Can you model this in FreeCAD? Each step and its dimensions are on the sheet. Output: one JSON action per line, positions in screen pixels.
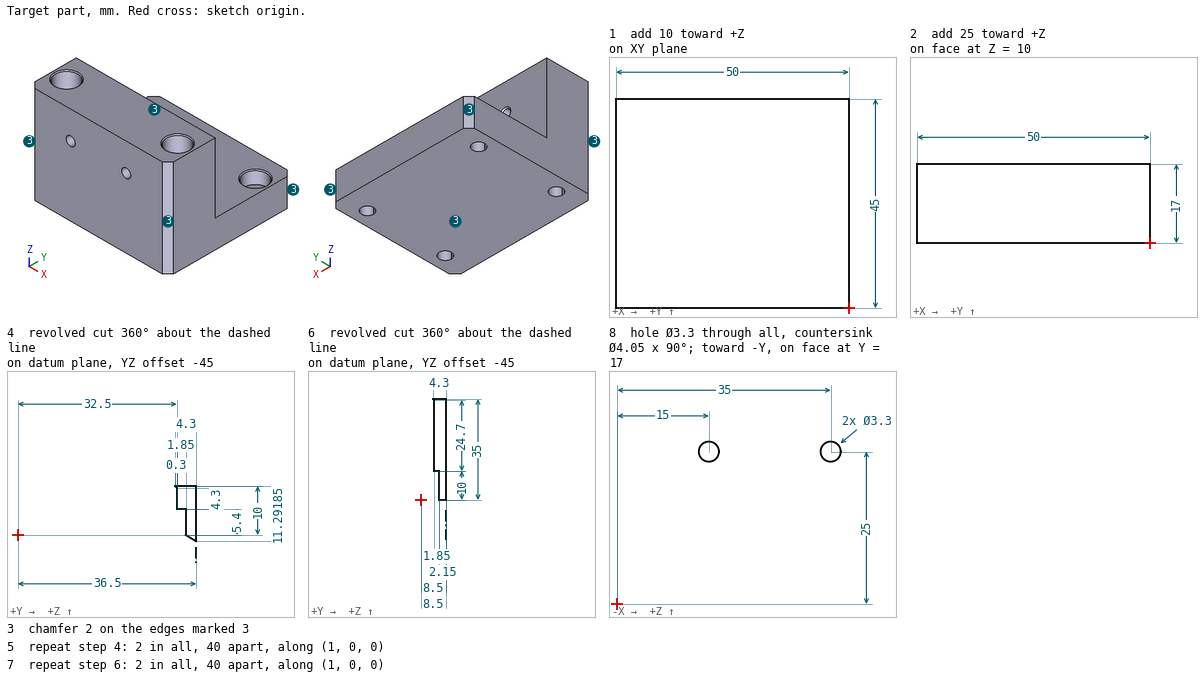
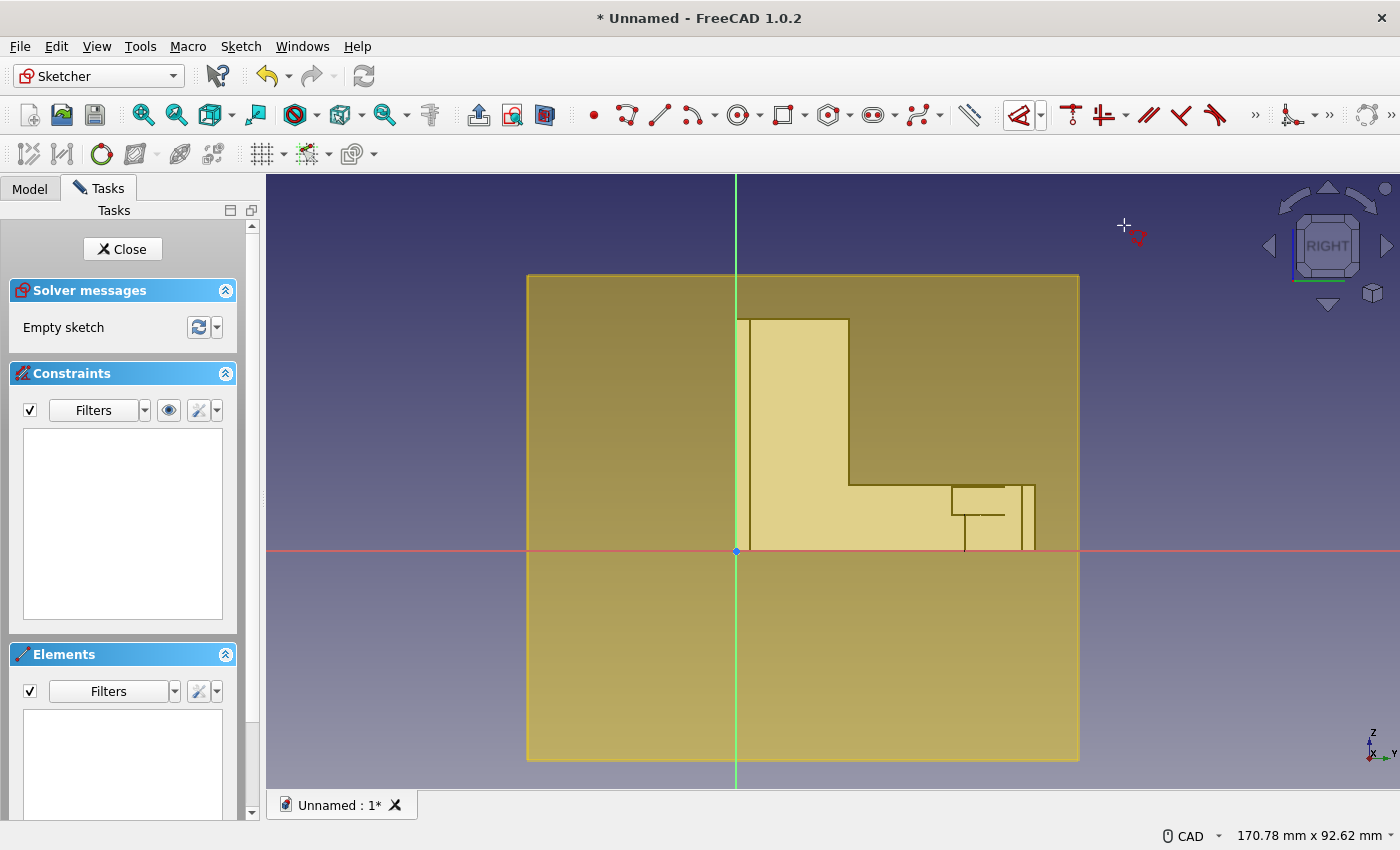
{"action": "left_click", "coordinate": [779, 551]}
{"action": "left_click", "coordinate": [793, 542]}
{"action": "left_click", "coordinate": [793, 319]}
{"action": "left_click", "coordinate": [764, 319]}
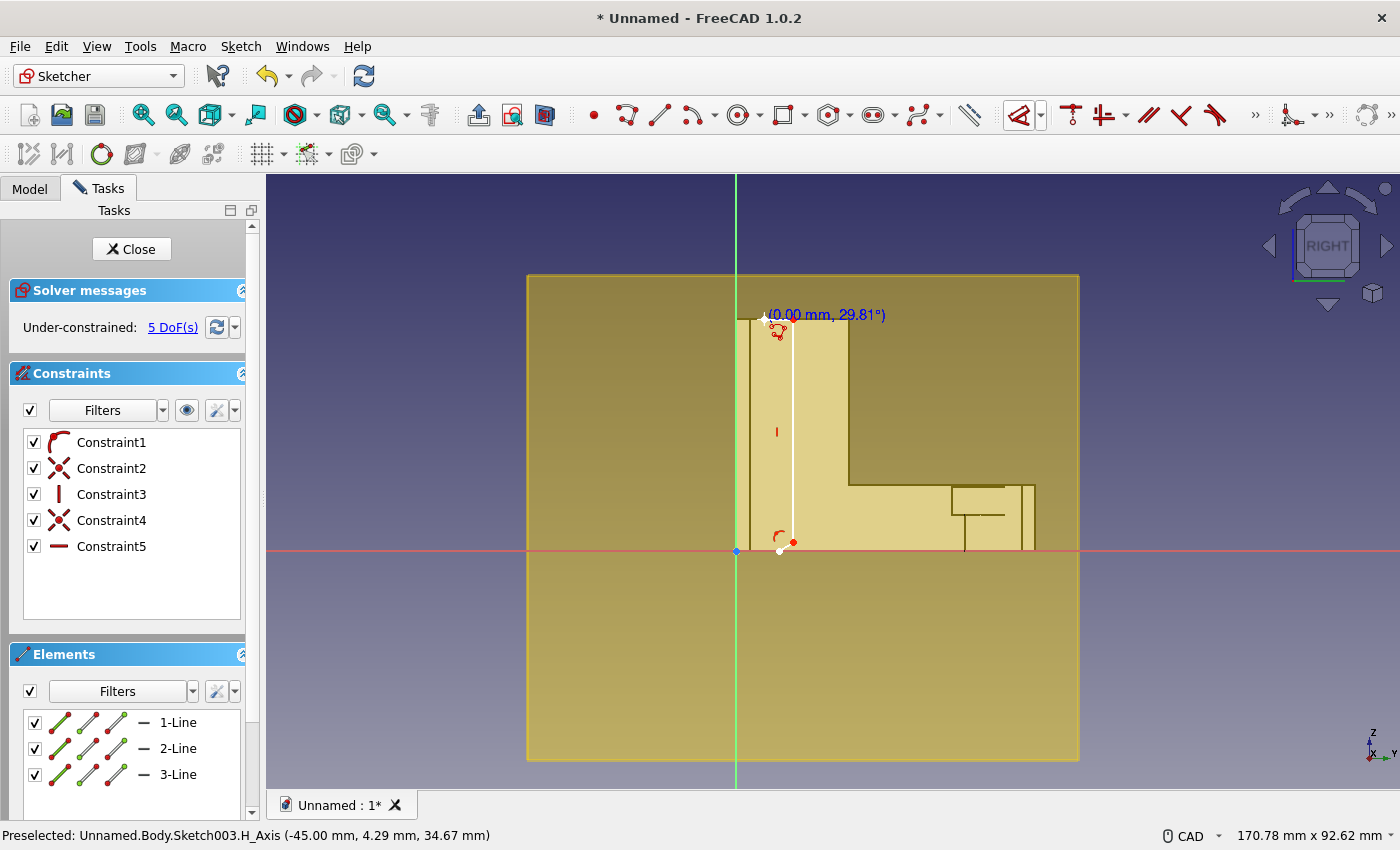
{"action": "scroll", "coordinate": [766, 321], "scroll_direction": "up", "scroll_amount": 11}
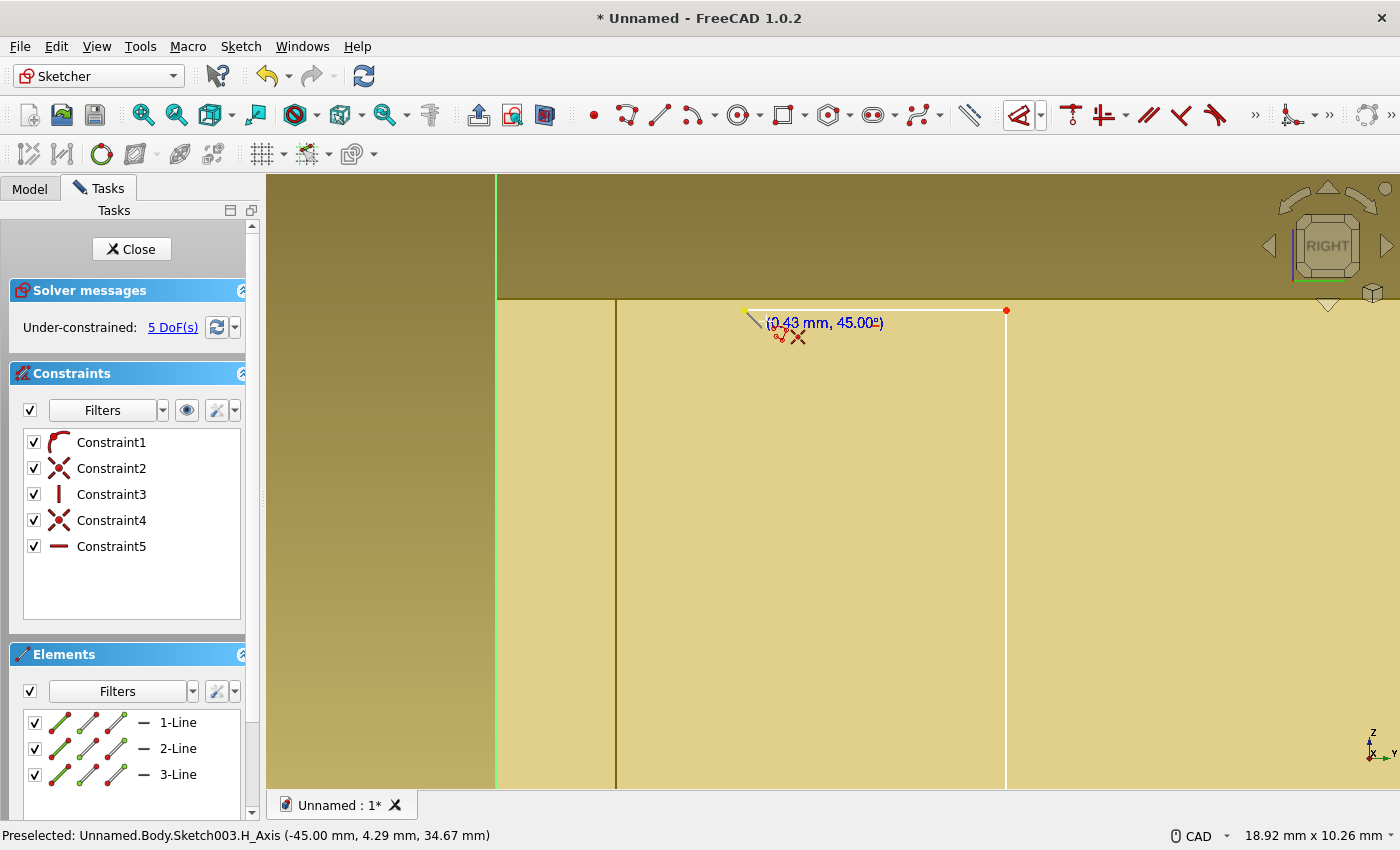
{"action": "left_click", "coordinate": [766, 317]}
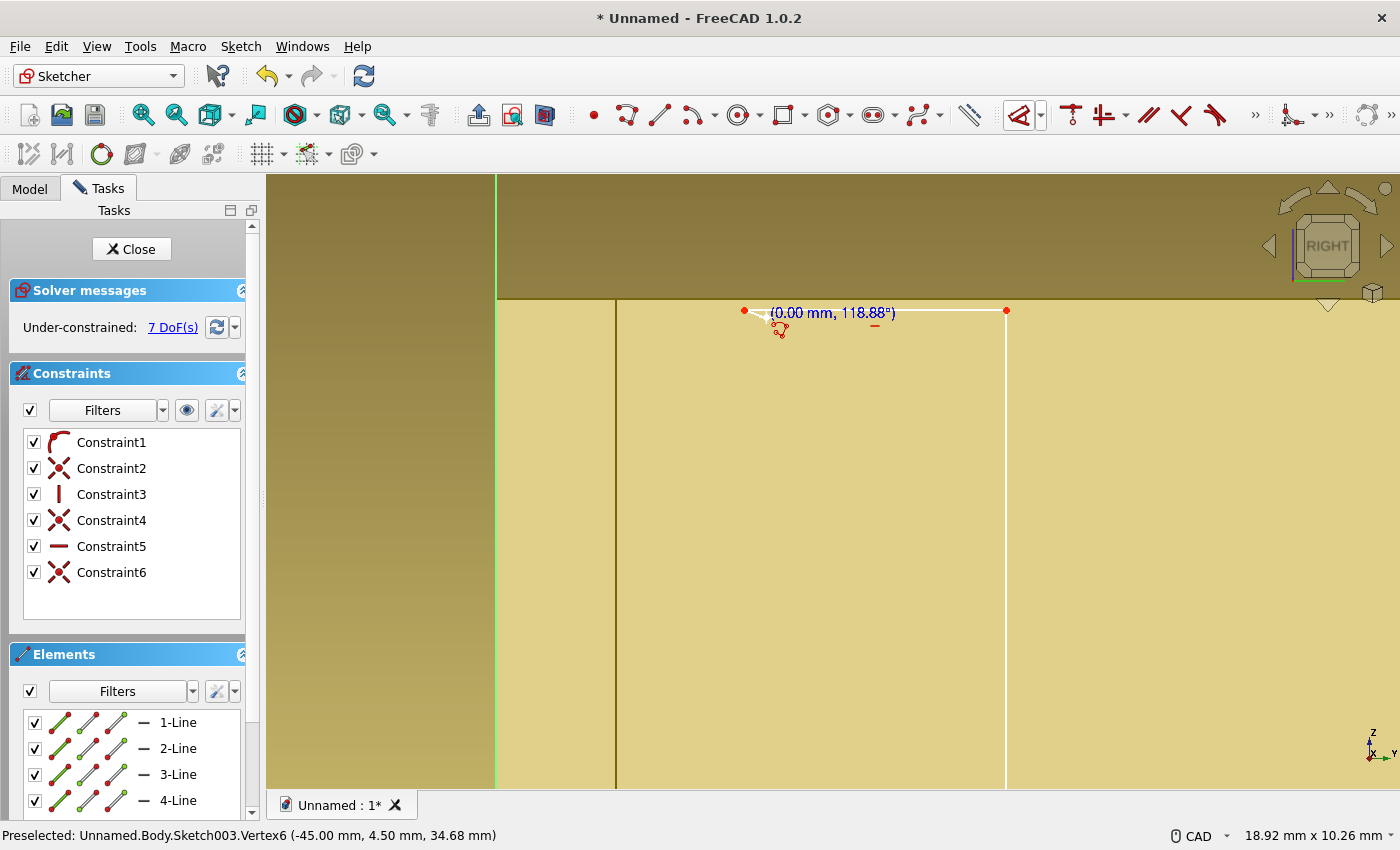
{"action": "scroll", "coordinate": [767, 280], "scroll_direction": "down", "scroll_amount": 10}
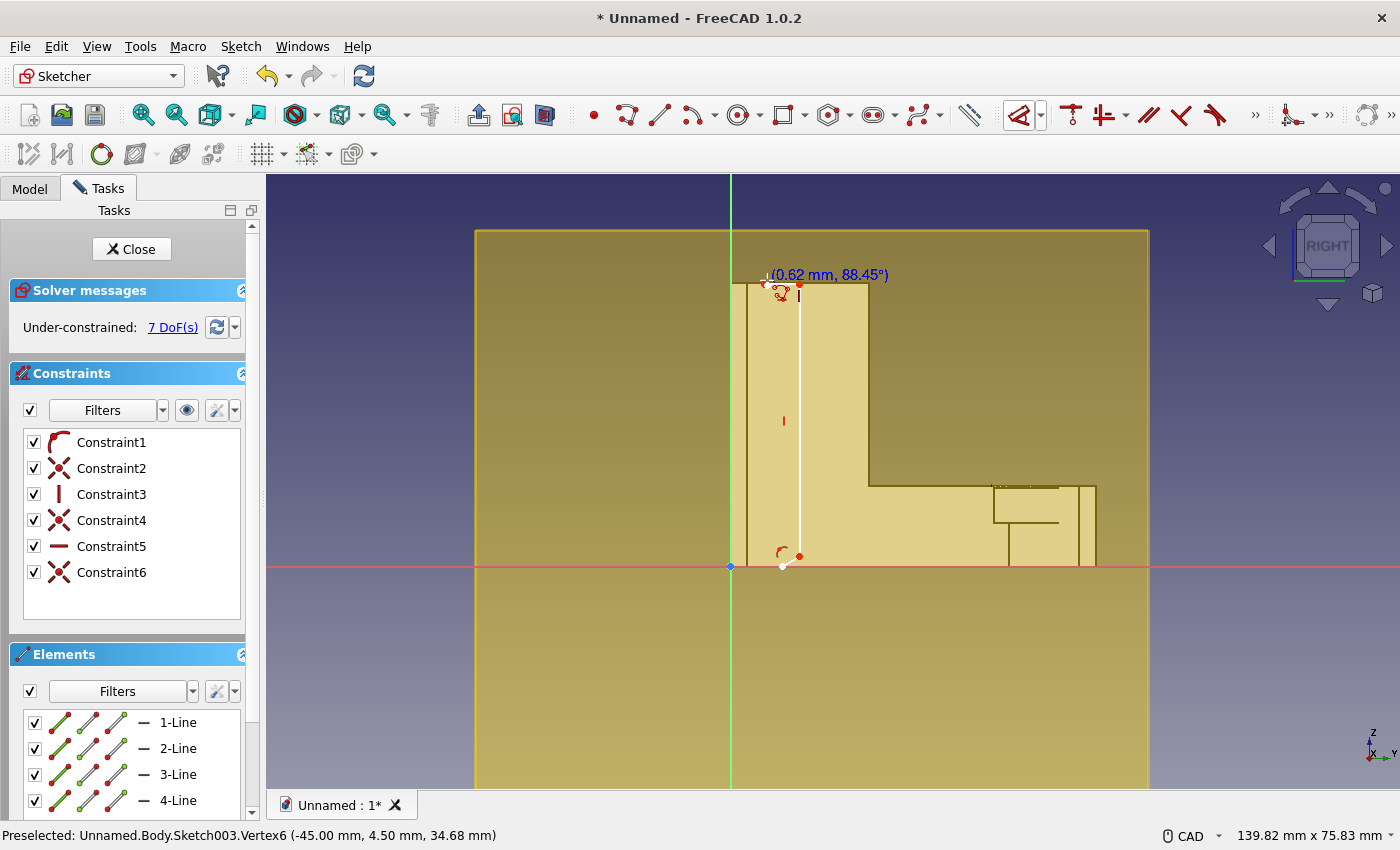
{"action": "left_click", "coordinate": [767, 486]}
{"action": "left_click", "coordinate": [782, 486]}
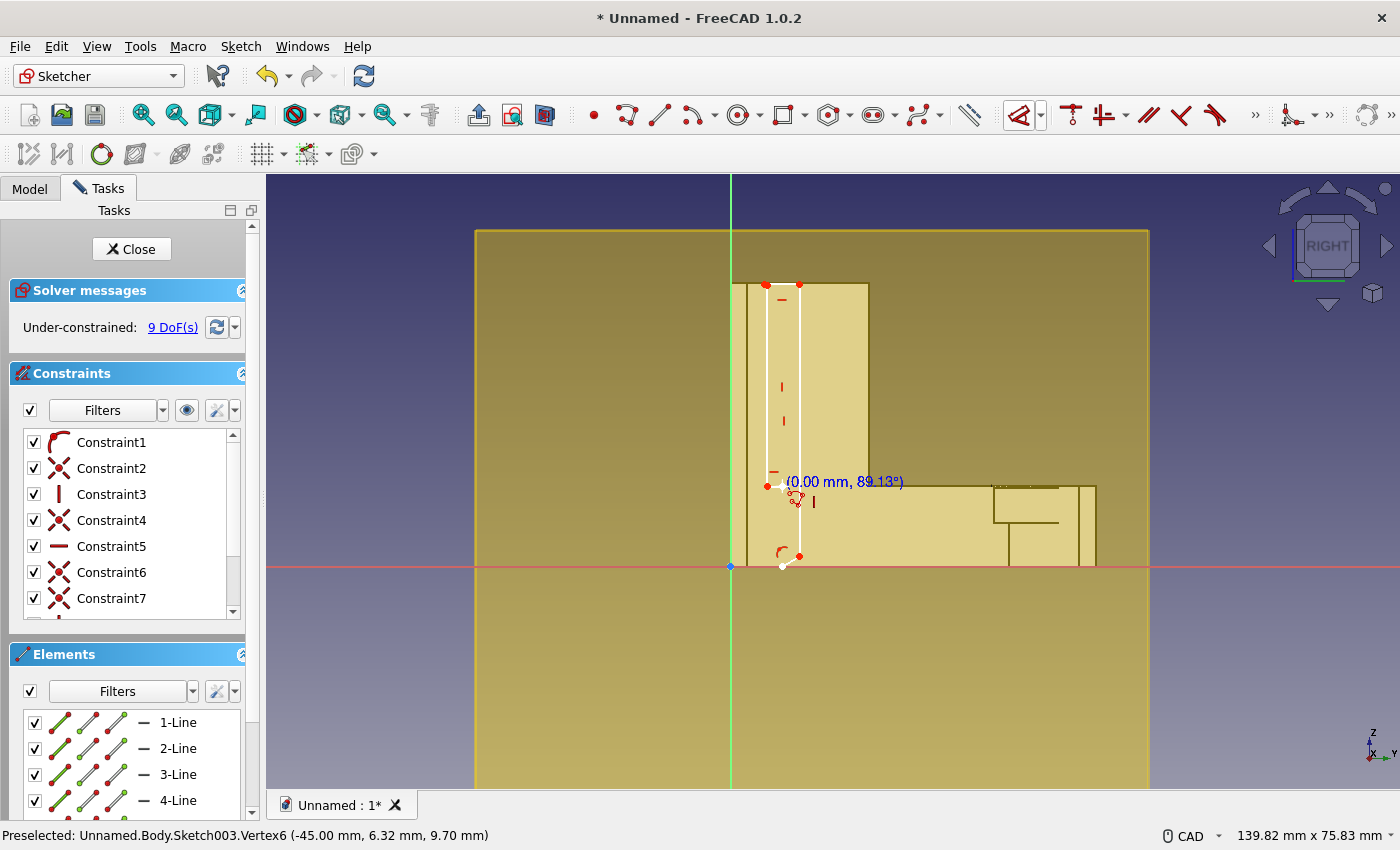
{"action": "scroll", "coordinate": [782, 567], "scroll_direction": "up", "scroll_amount": 3}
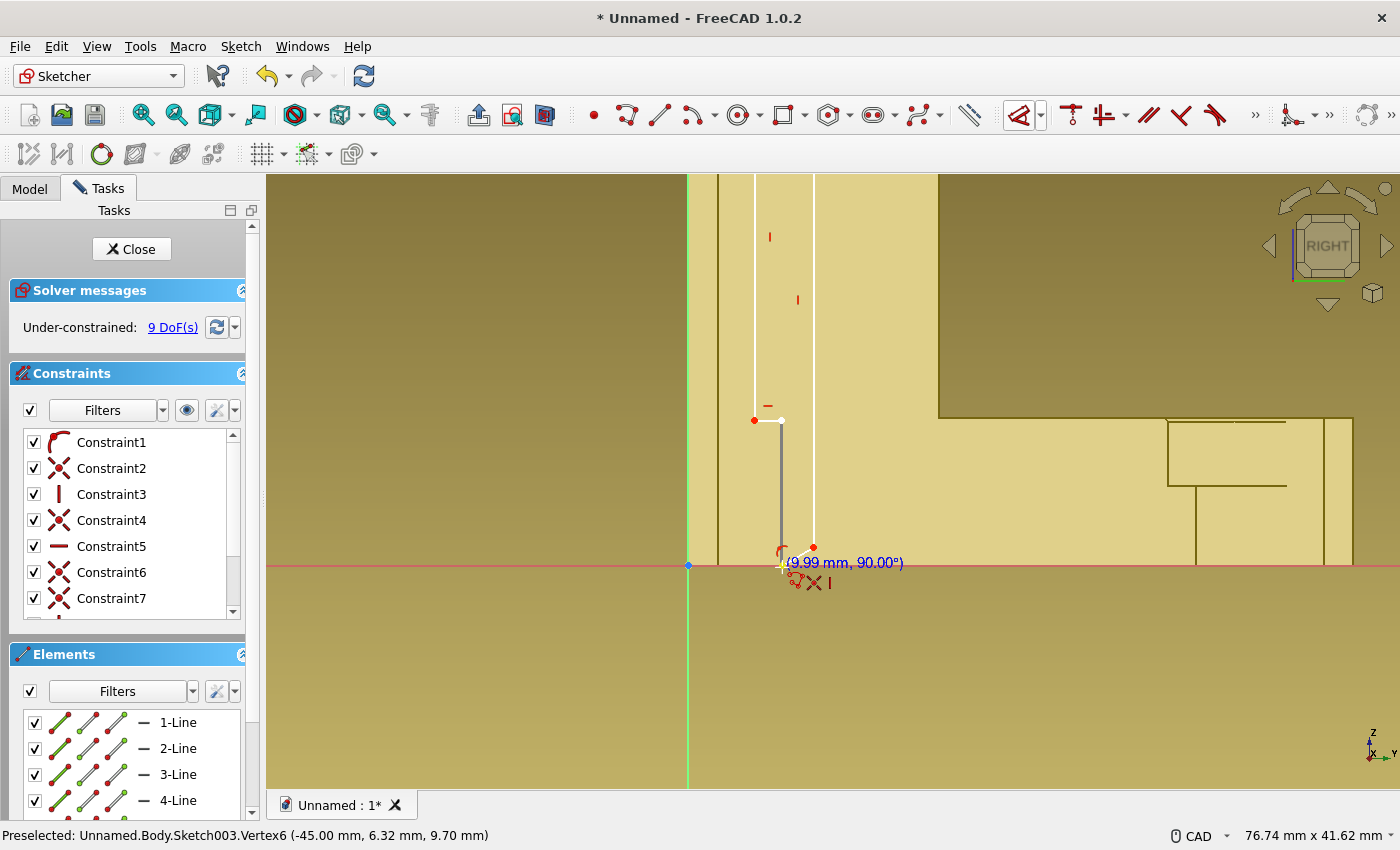
{"action": "left_click", "coordinate": [783, 566]}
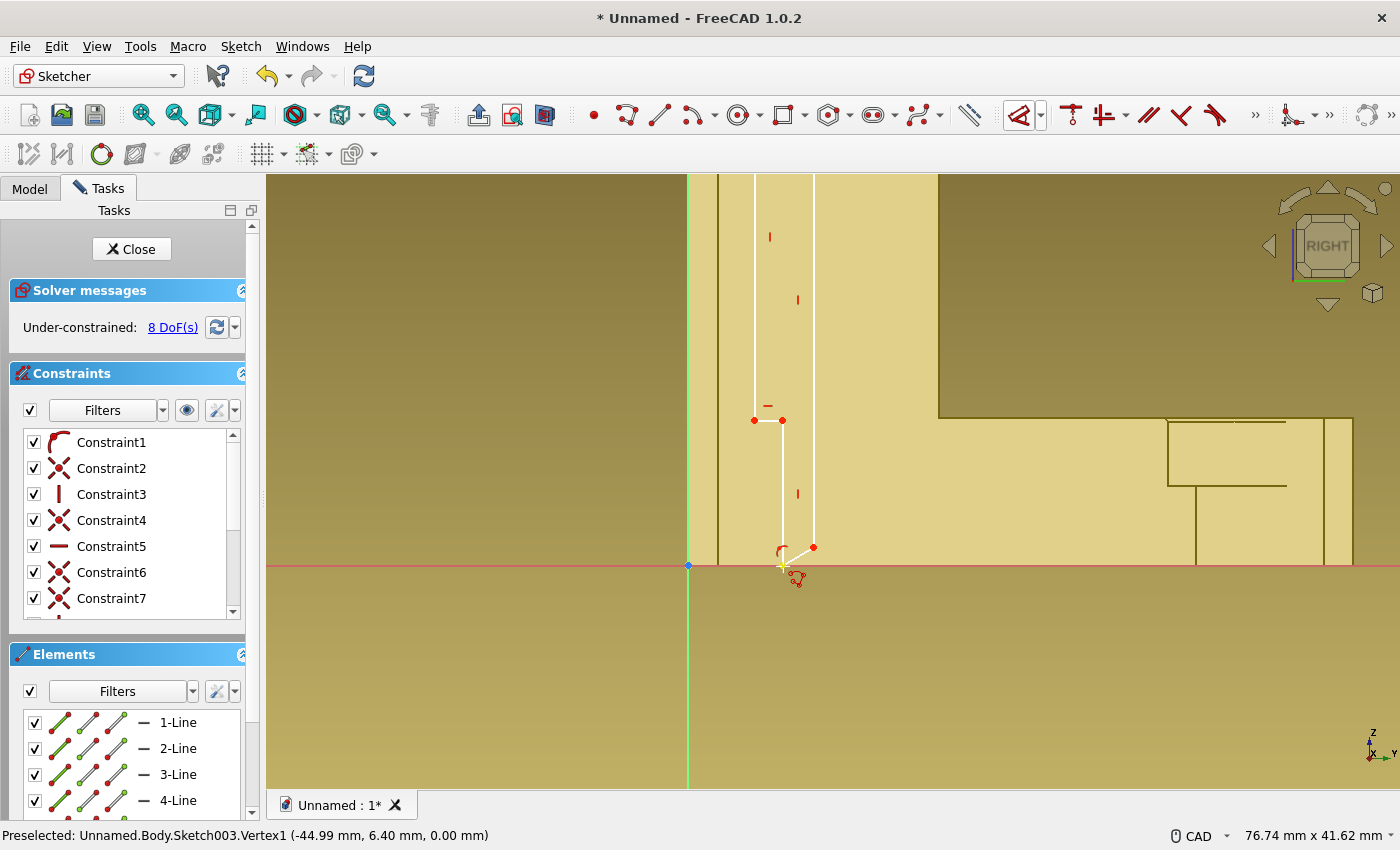
{"action": "key", "text": "g l"}